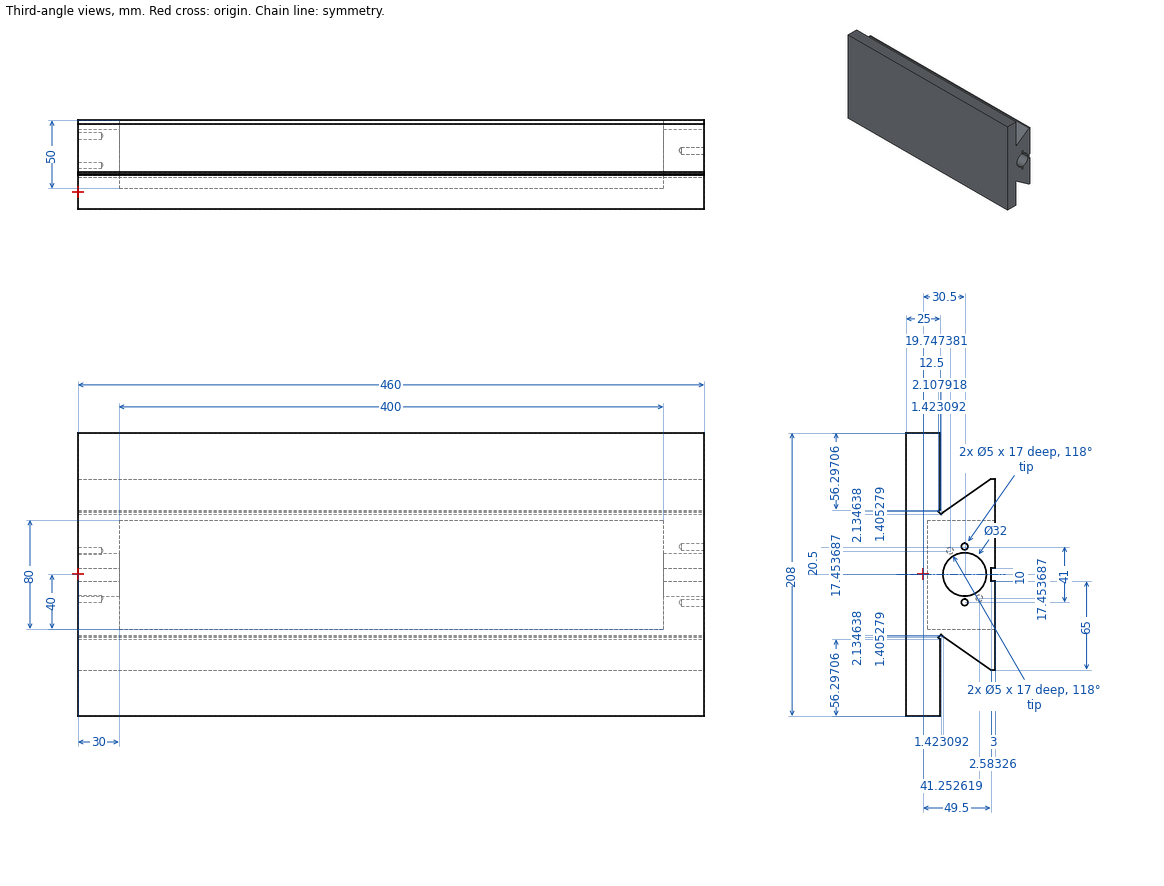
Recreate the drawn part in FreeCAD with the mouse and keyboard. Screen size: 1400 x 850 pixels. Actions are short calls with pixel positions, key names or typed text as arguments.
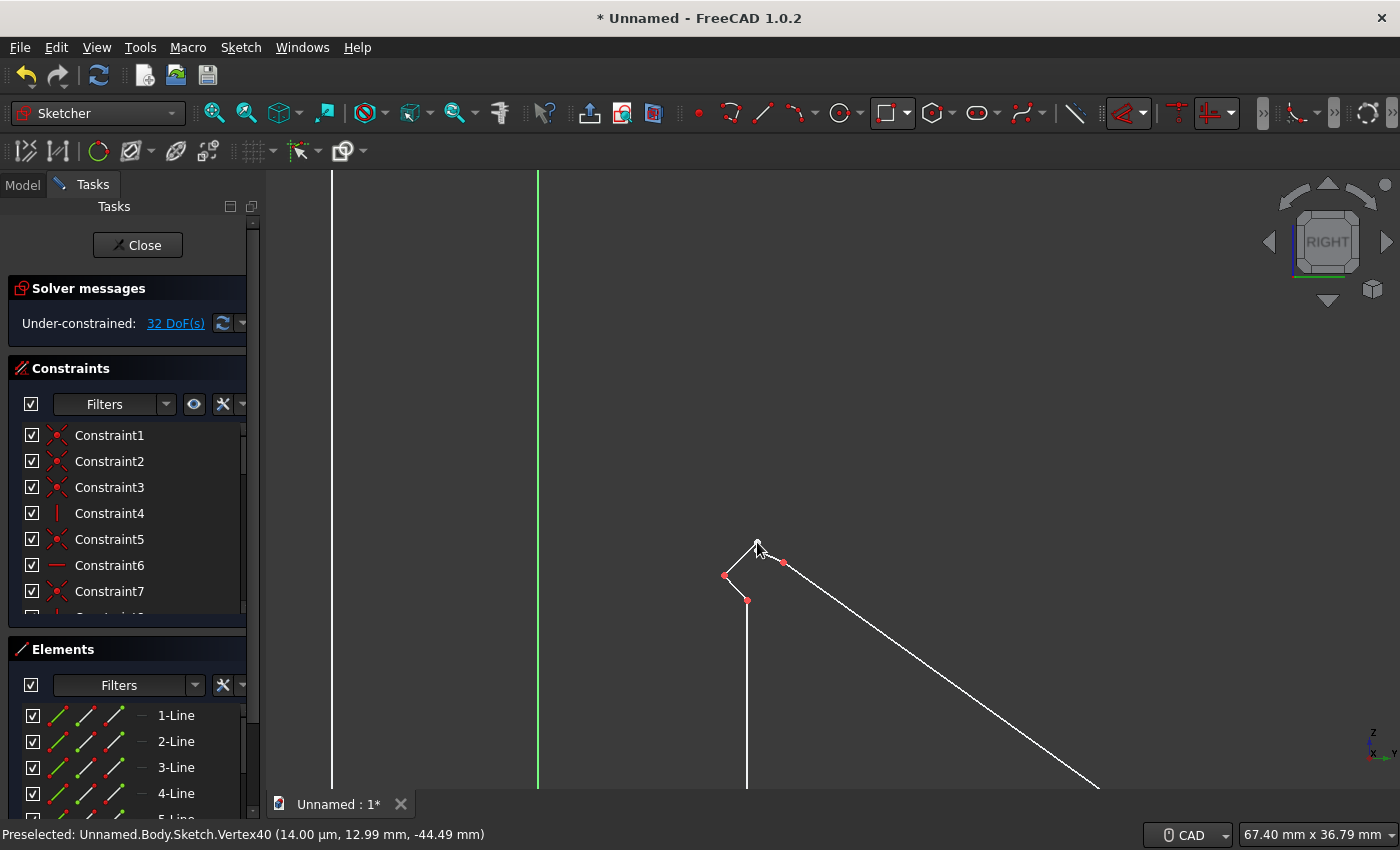
scroll(751, 565, down, 11)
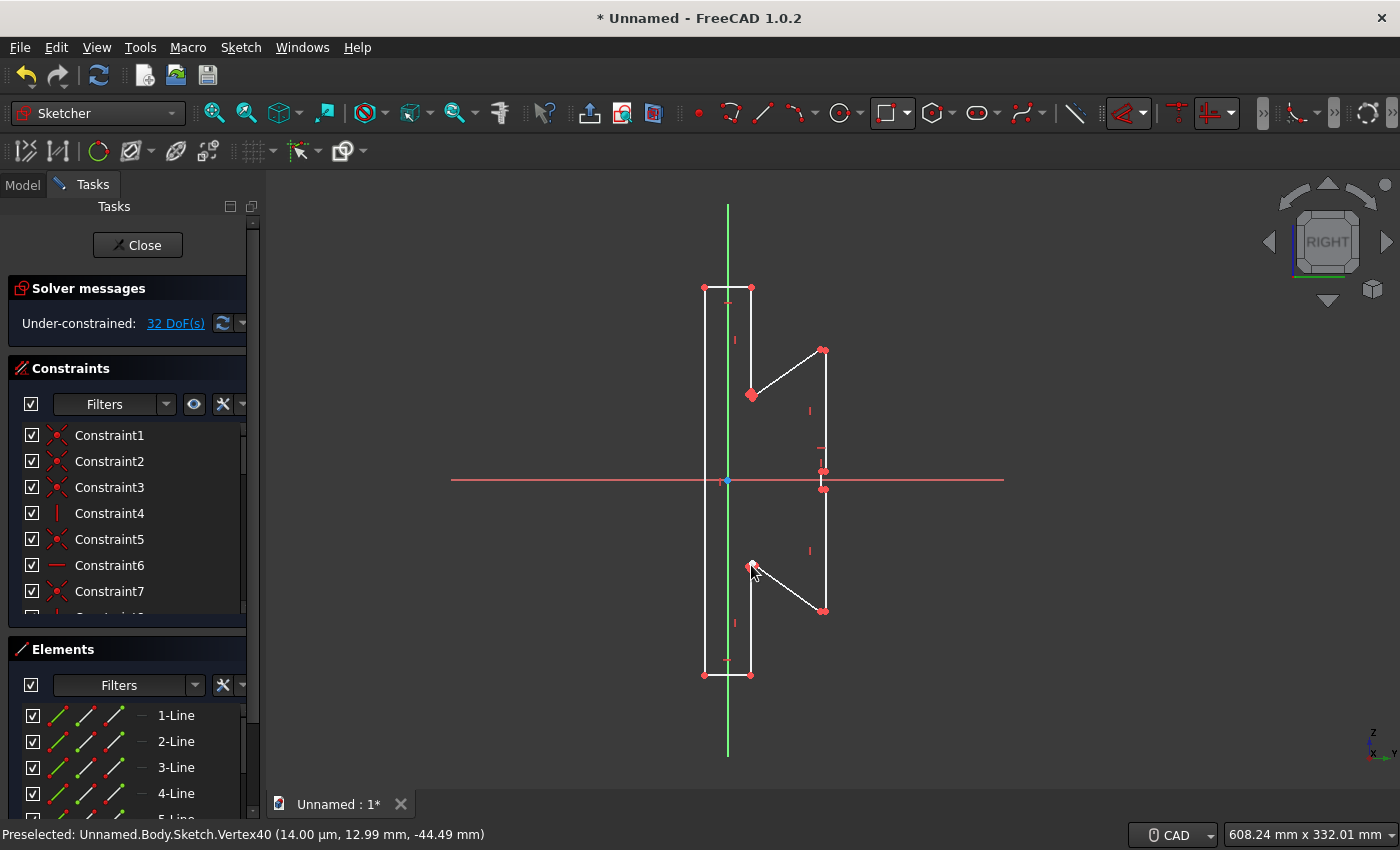
scroll(822, 612, up, 11)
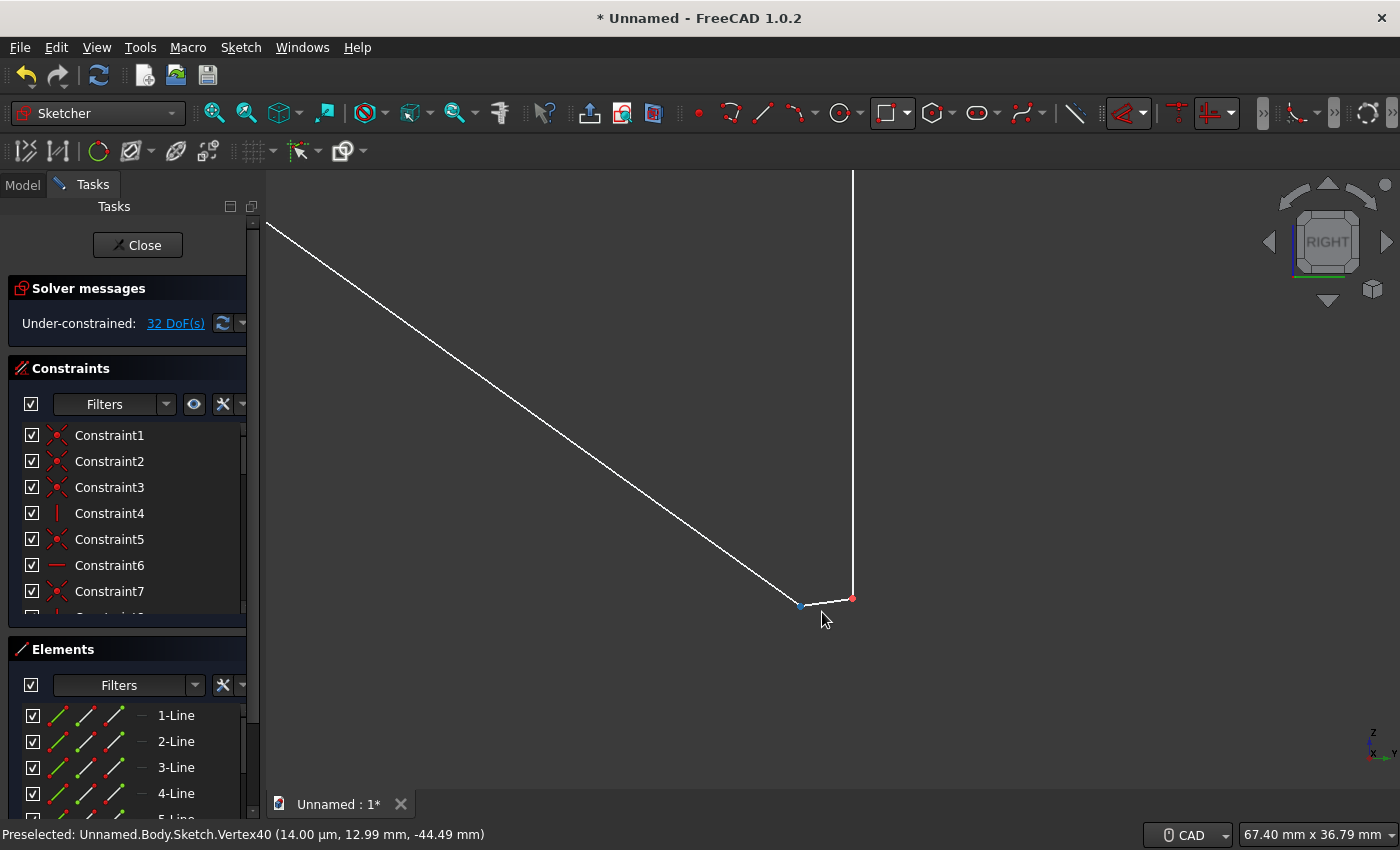
click(816, 604)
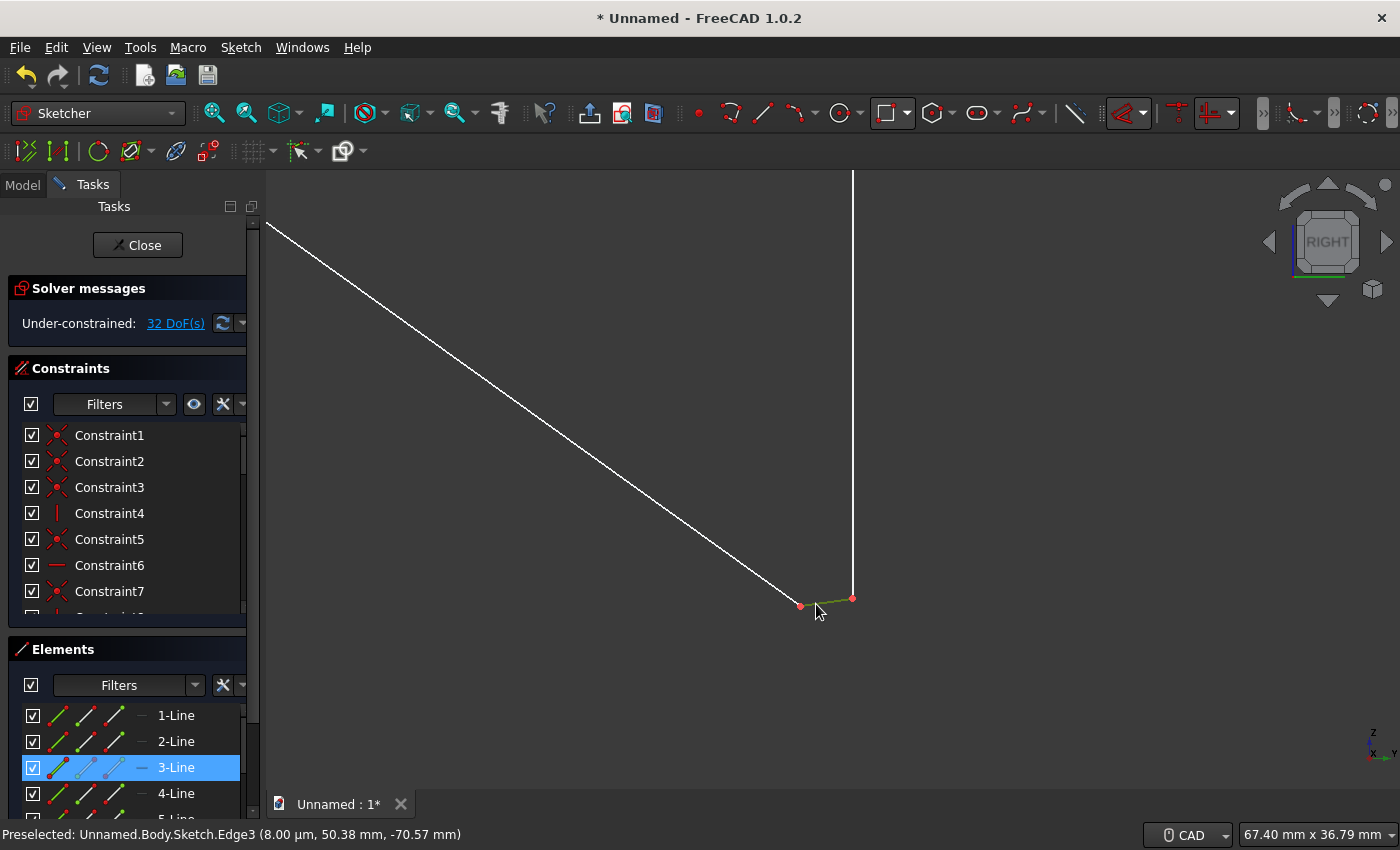
click(1234, 114)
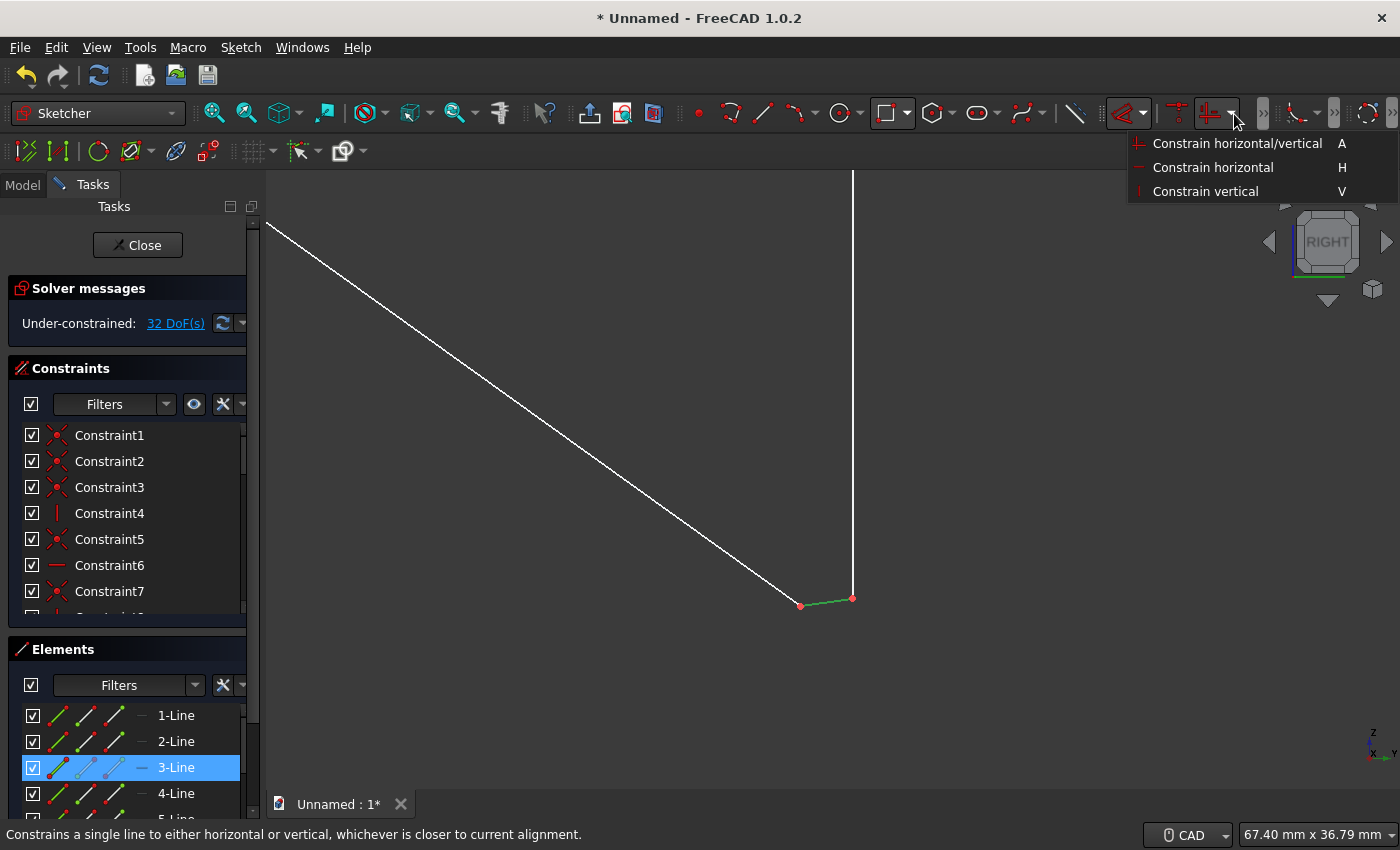
click(1263, 167)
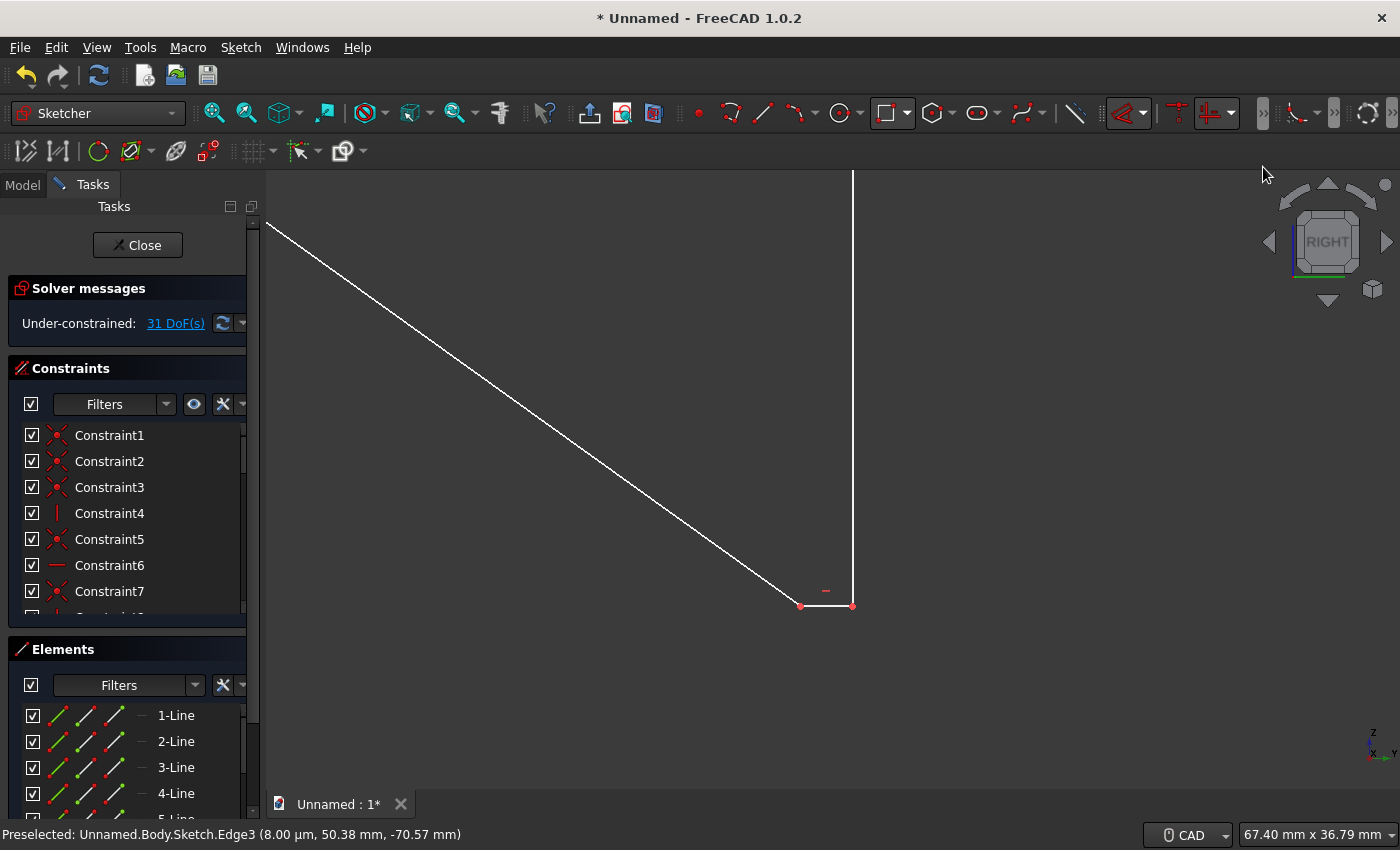
scroll(822, 612, down, 11)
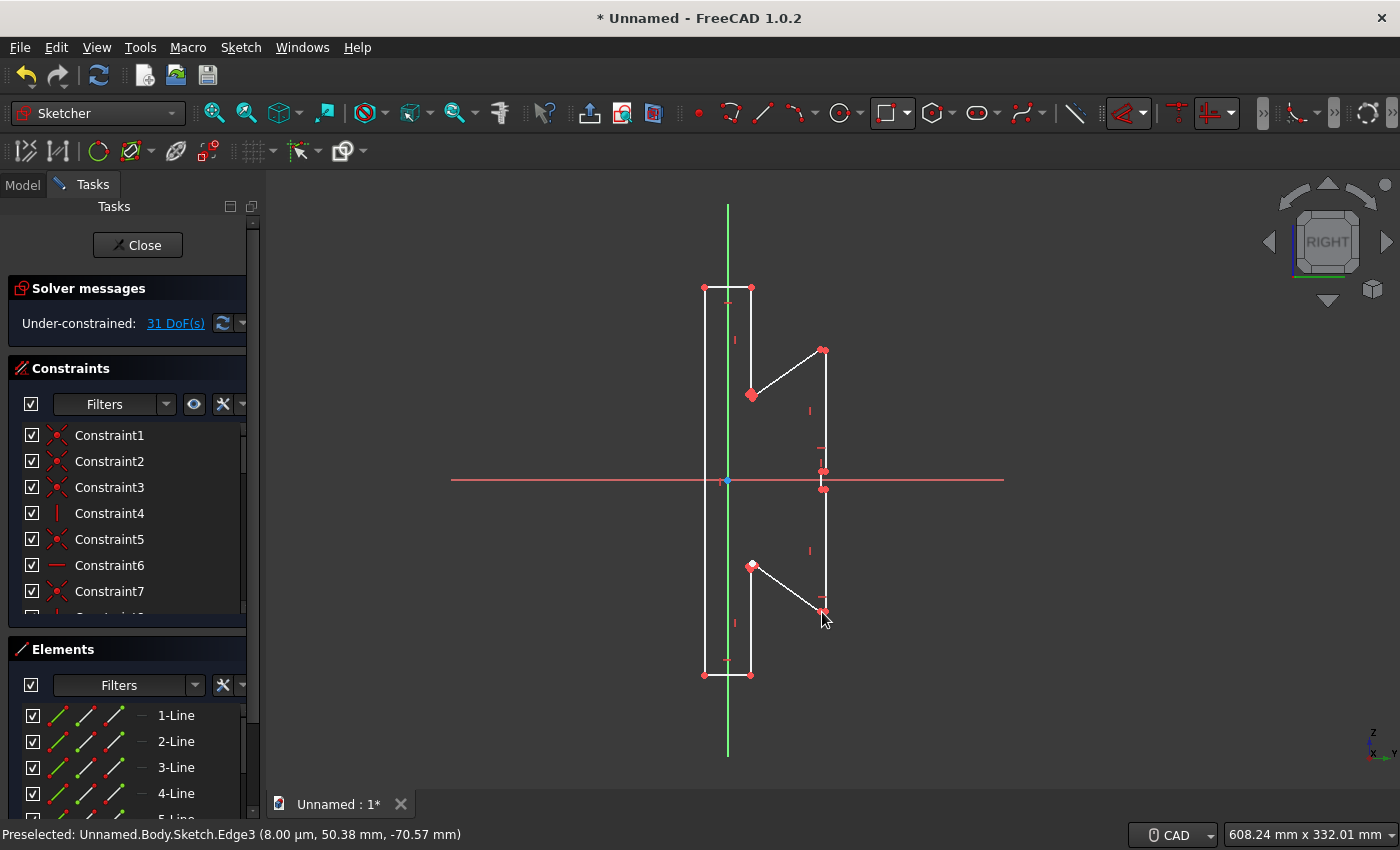
scroll(824, 350, up, 11)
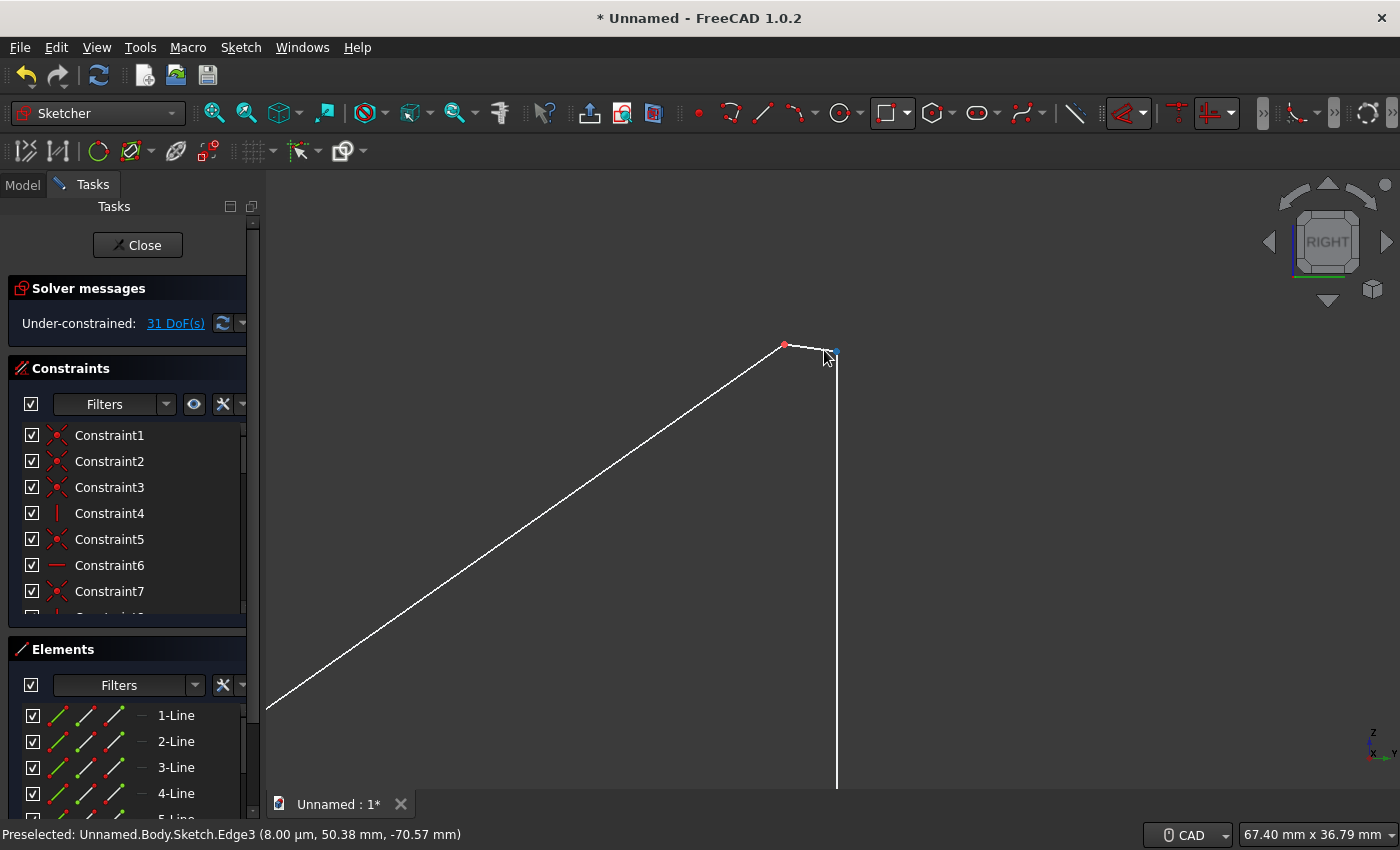
click(821, 349)